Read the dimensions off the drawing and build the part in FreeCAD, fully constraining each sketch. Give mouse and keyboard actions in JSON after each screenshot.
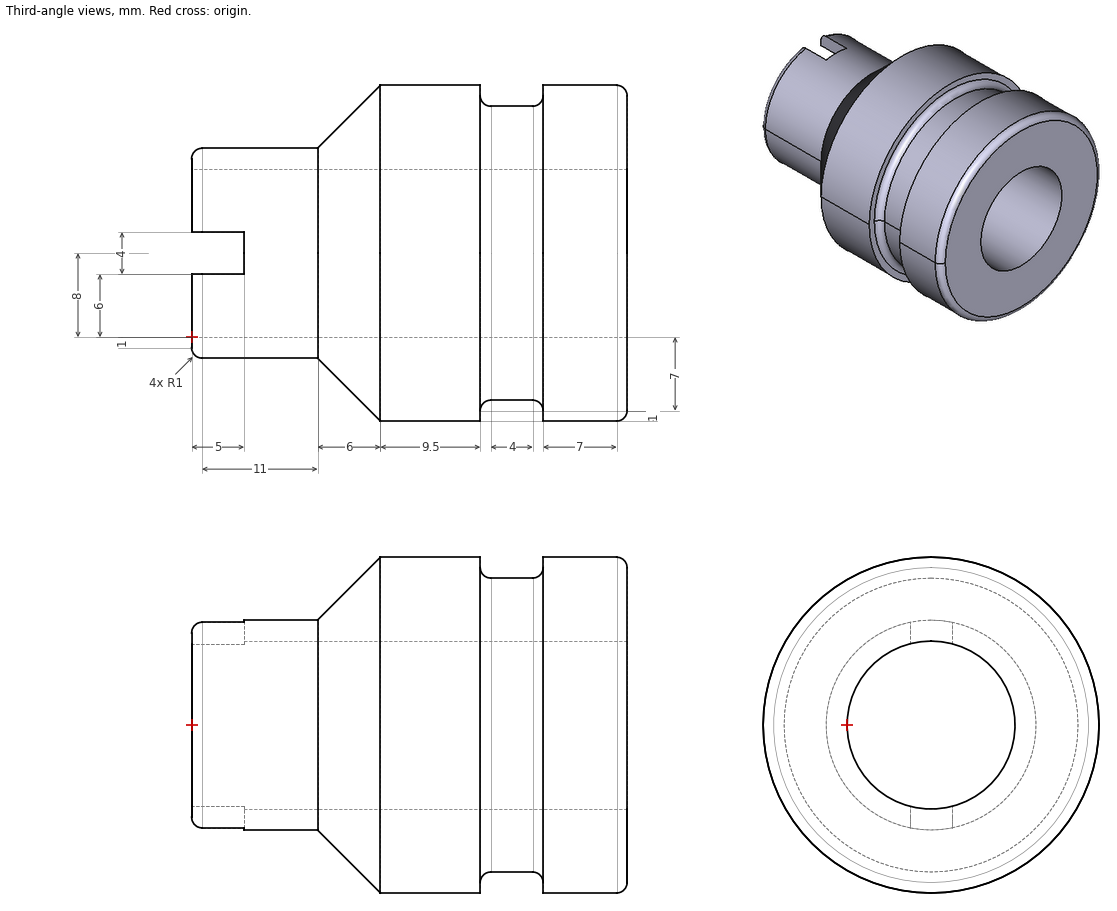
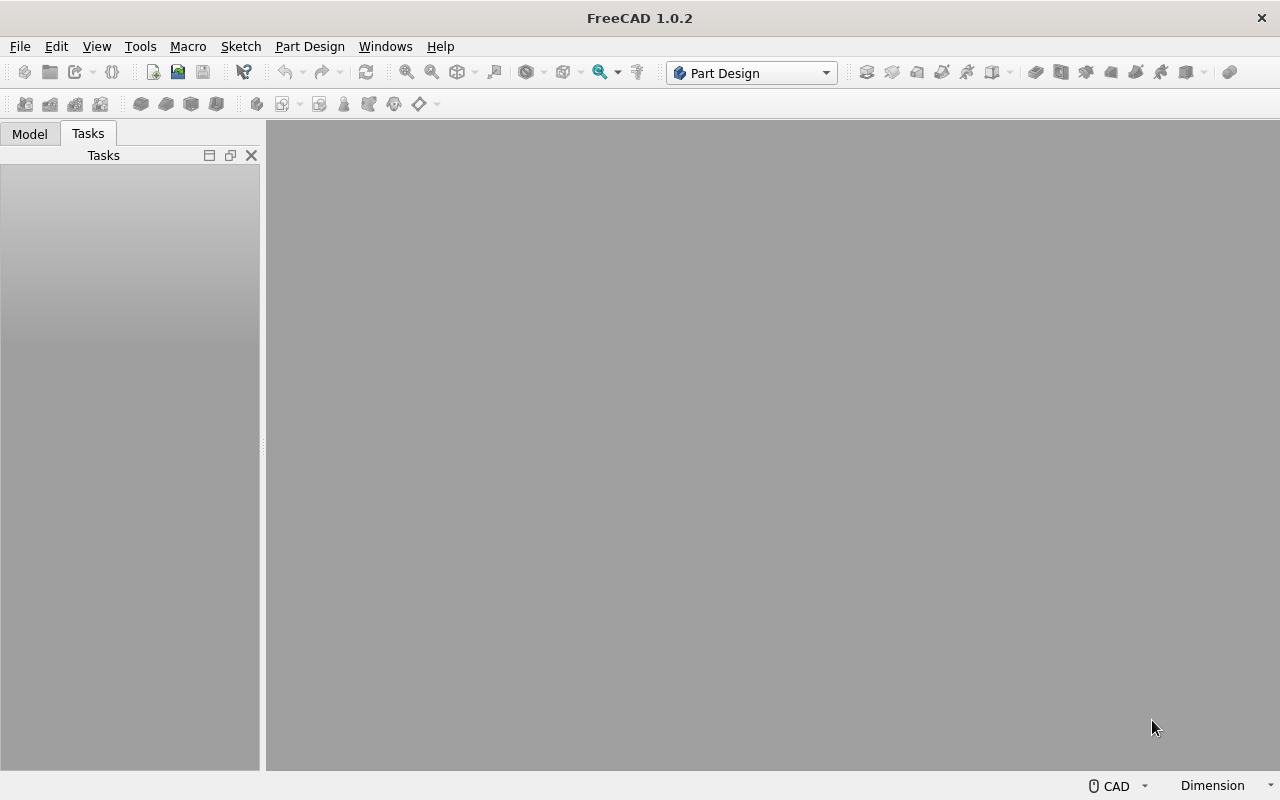
{"action": "key", "text": "ctrl+n"}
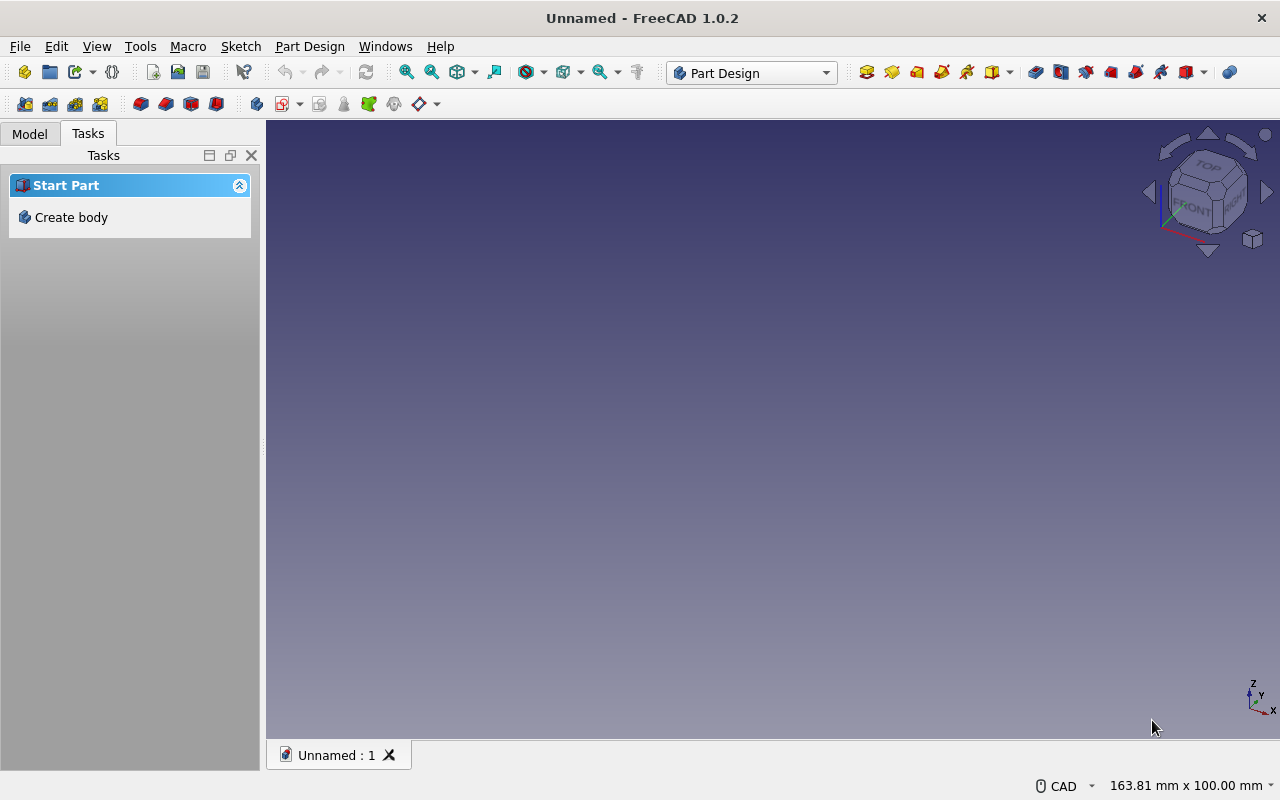
{"action": "left_click", "coordinate": [282, 104]}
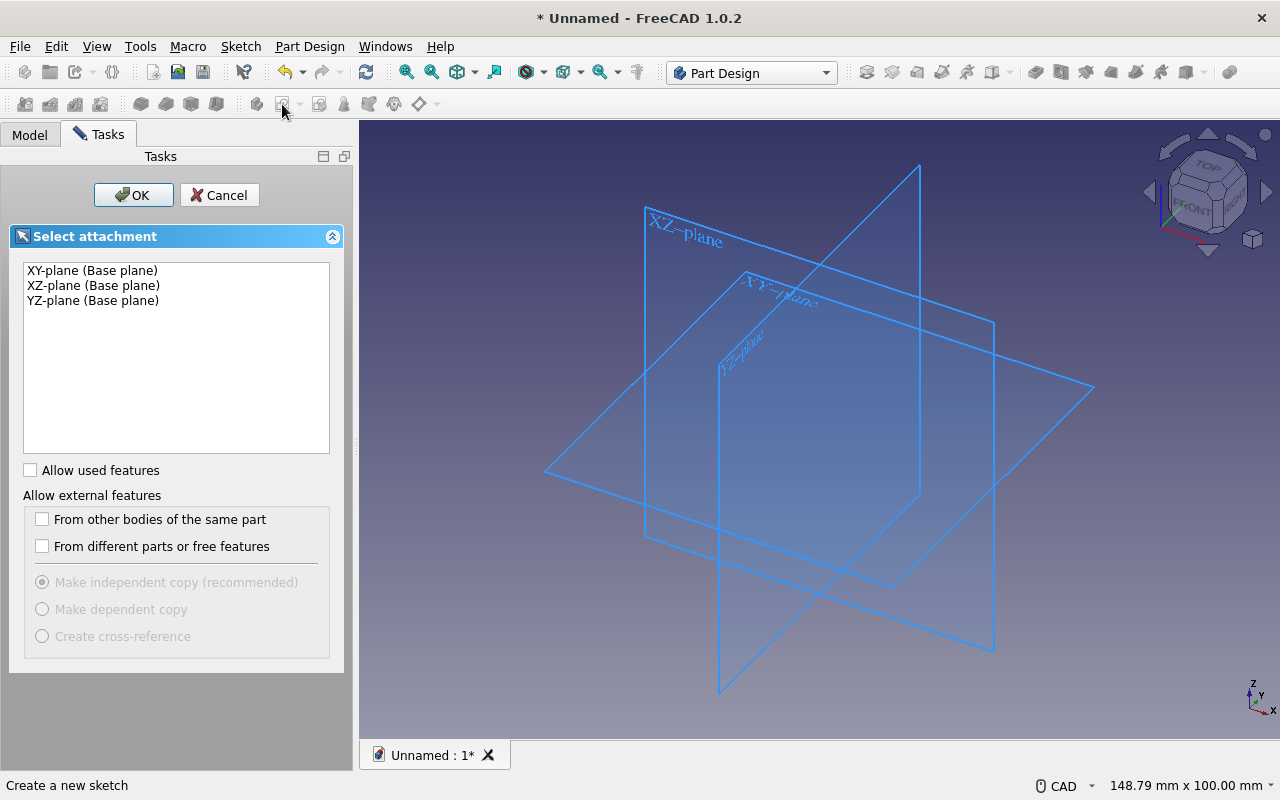
{"action": "left_click", "coordinate": [84, 270]}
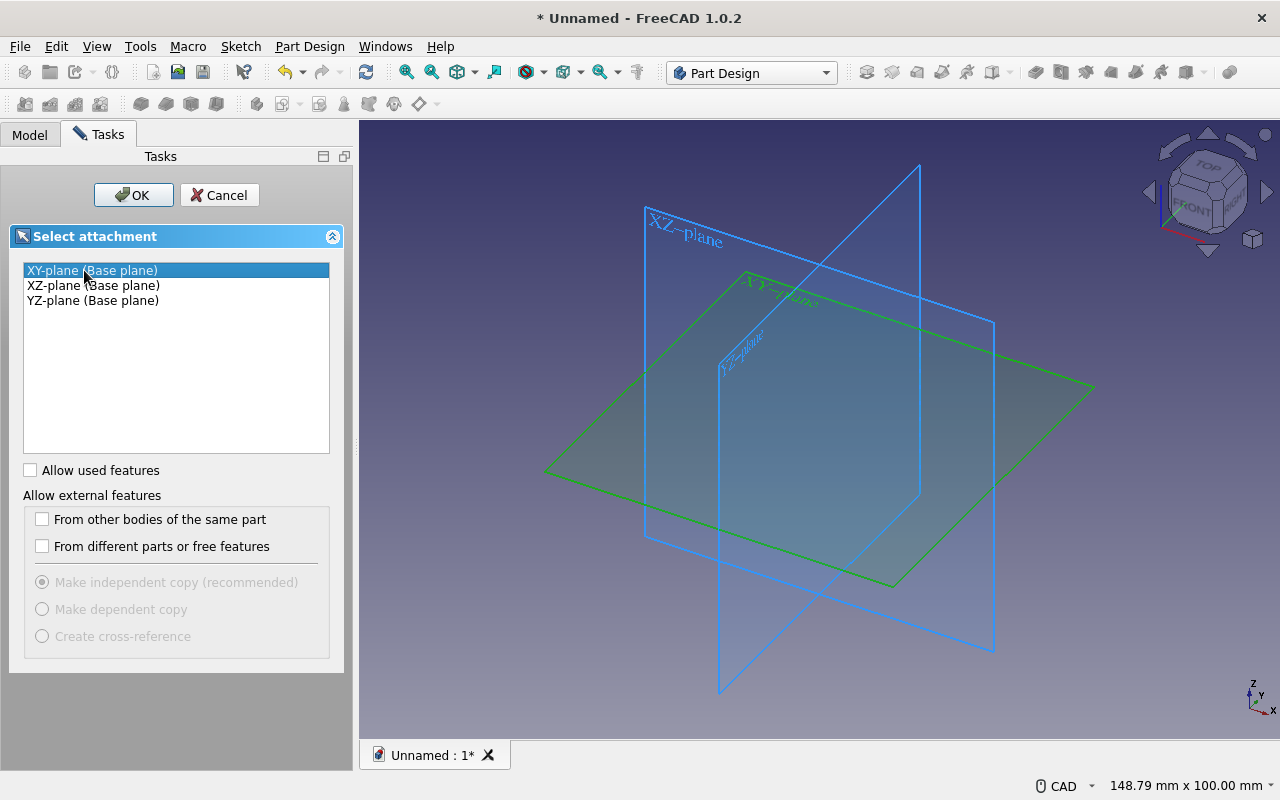
{"action": "left_click", "coordinate": [134, 195]}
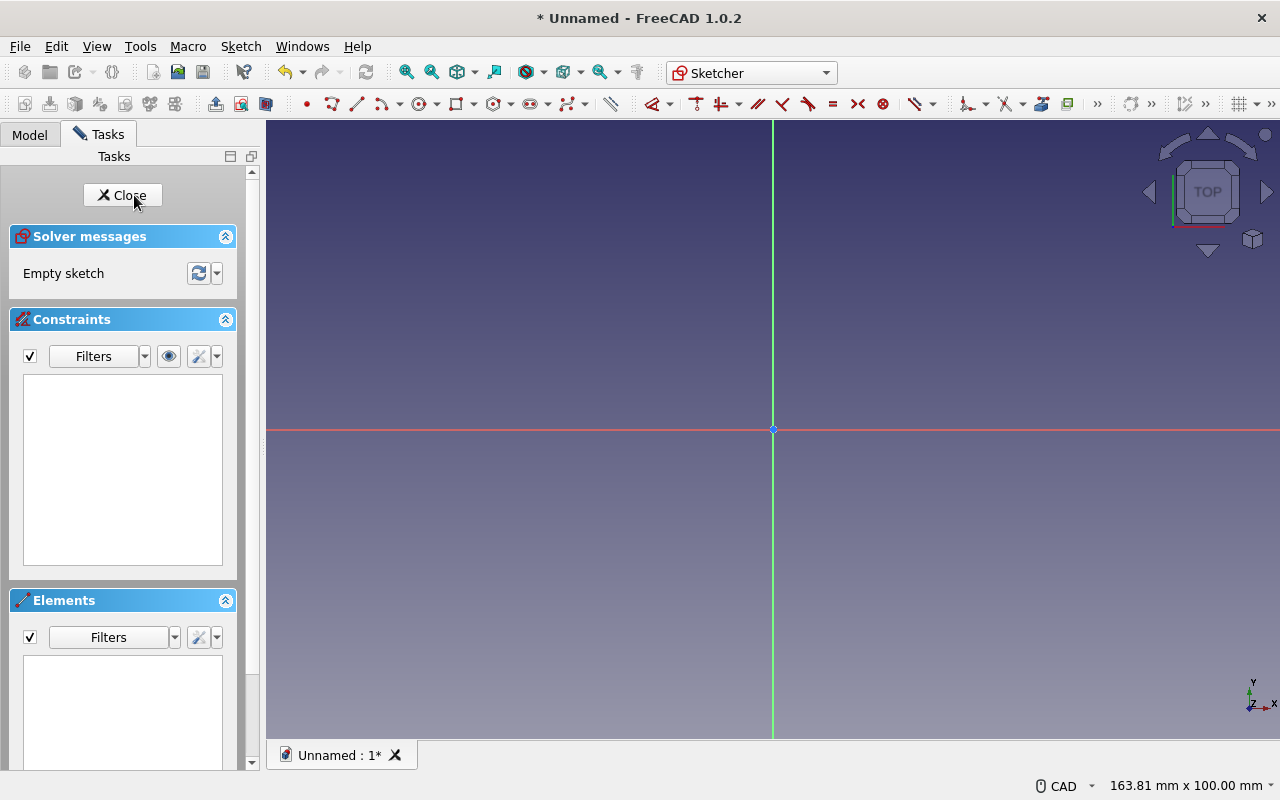
{"action": "scroll", "coordinate": [1115, 430], "scroll_direction": "up", "scroll_amount": 3}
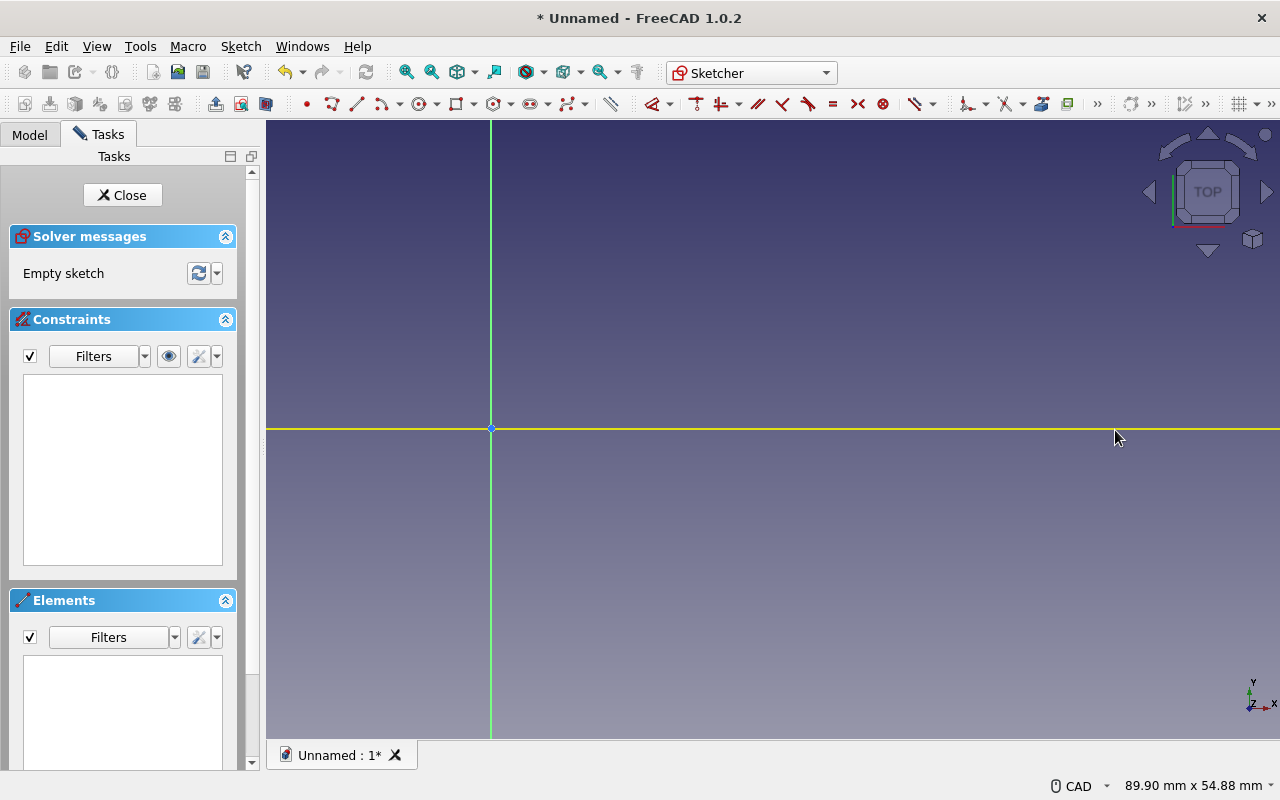
{"action": "left_click", "coordinate": [332, 104]}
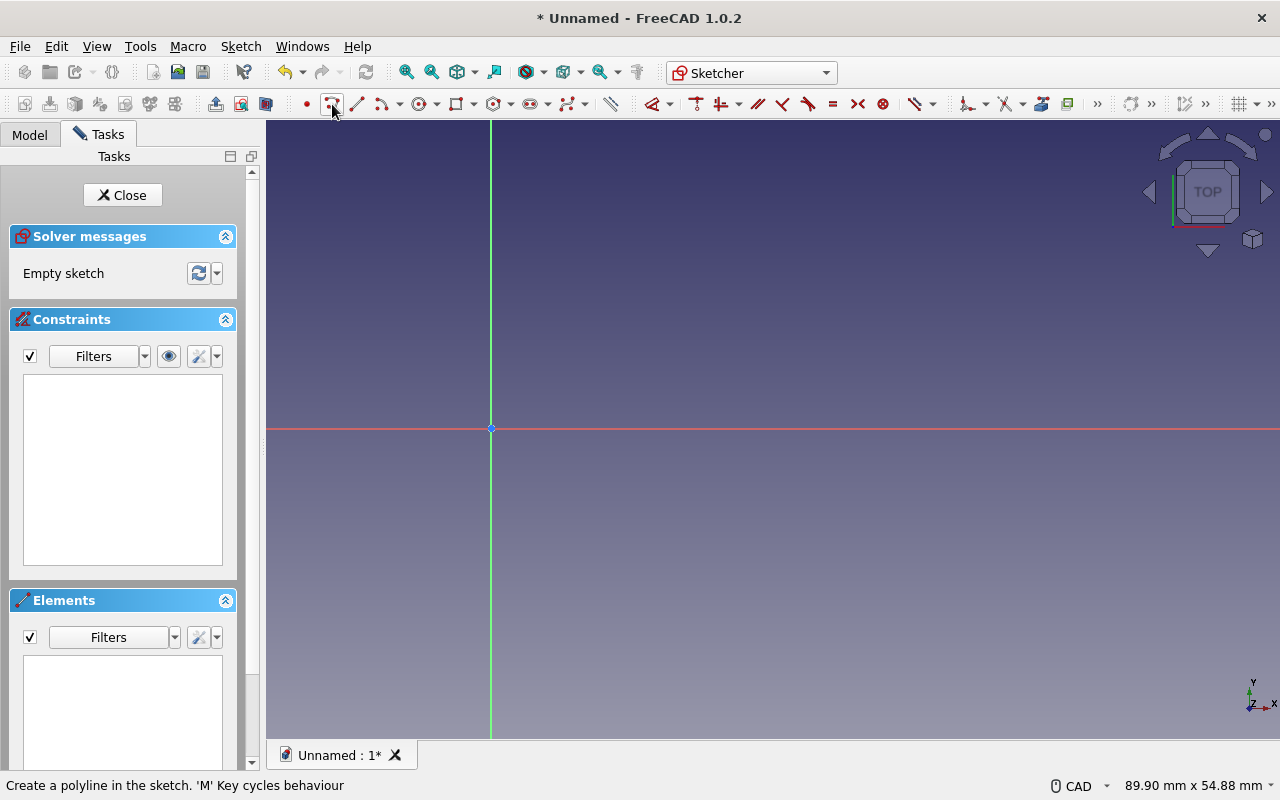
{"action": "scroll", "coordinate": [502, 451], "scroll_direction": "up", "scroll_amount": 2}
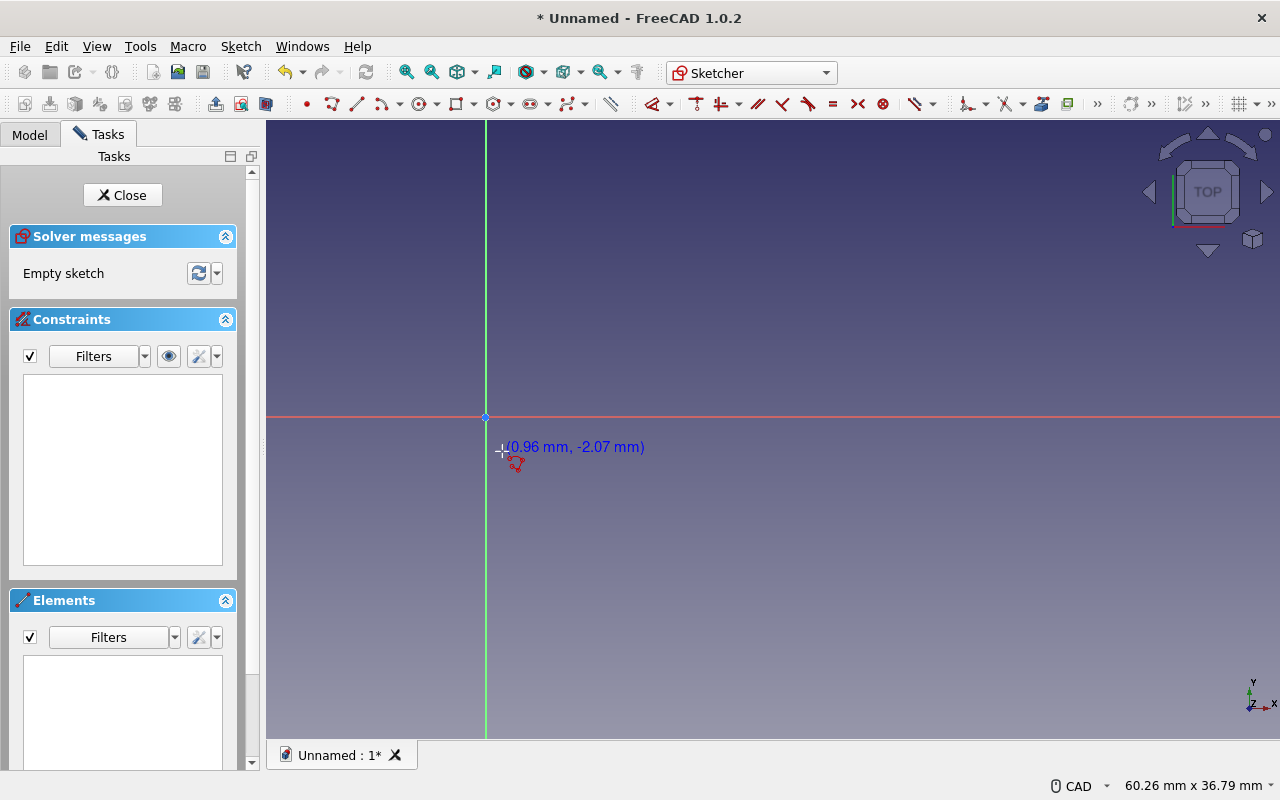
{"action": "left_click", "coordinate": [503, 451]}
{"action": "left_click", "coordinate": [688, 451]}
{"action": "left_click", "coordinate": [789, 552]}
{"action": "left_click", "coordinate": [948, 552]}
{"action": "left_click", "coordinate": [948, 535]}
{"action": "right_click", "coordinate": [948, 535]}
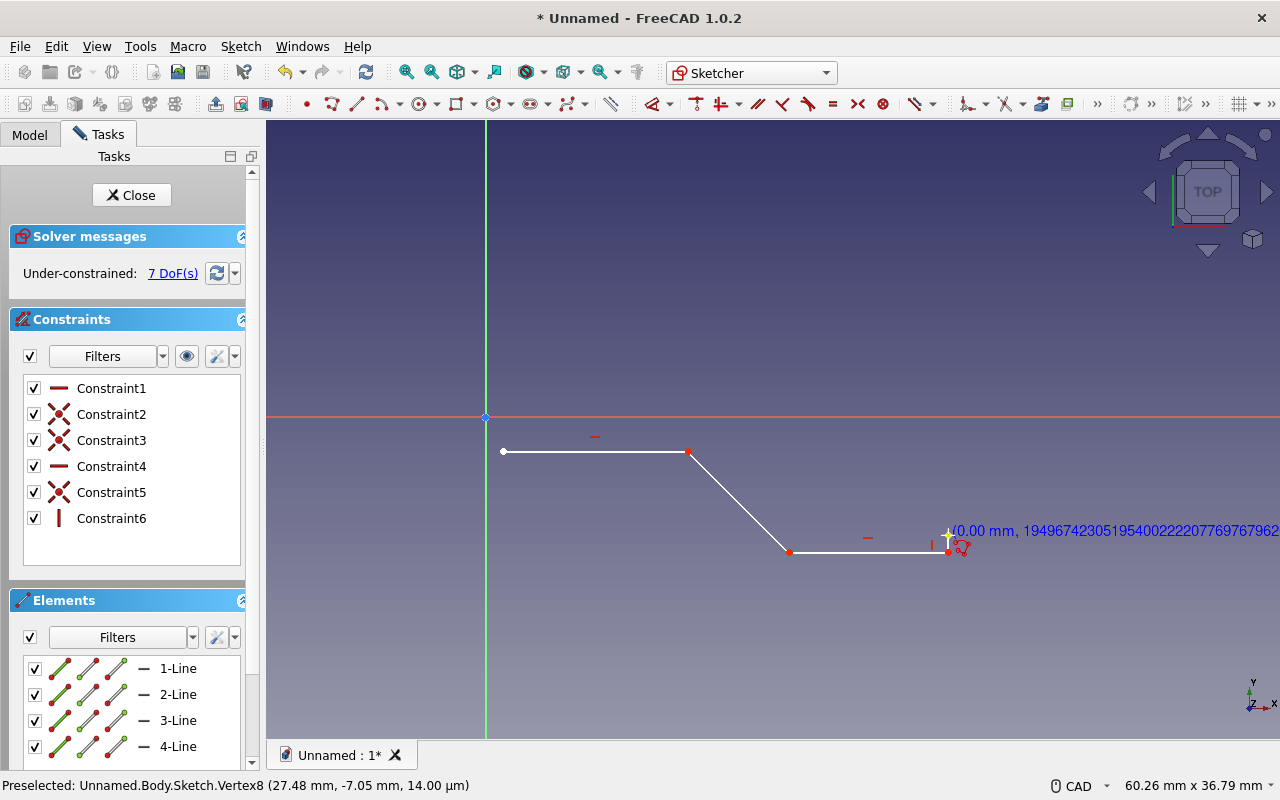
{"action": "key", "text": "g l"}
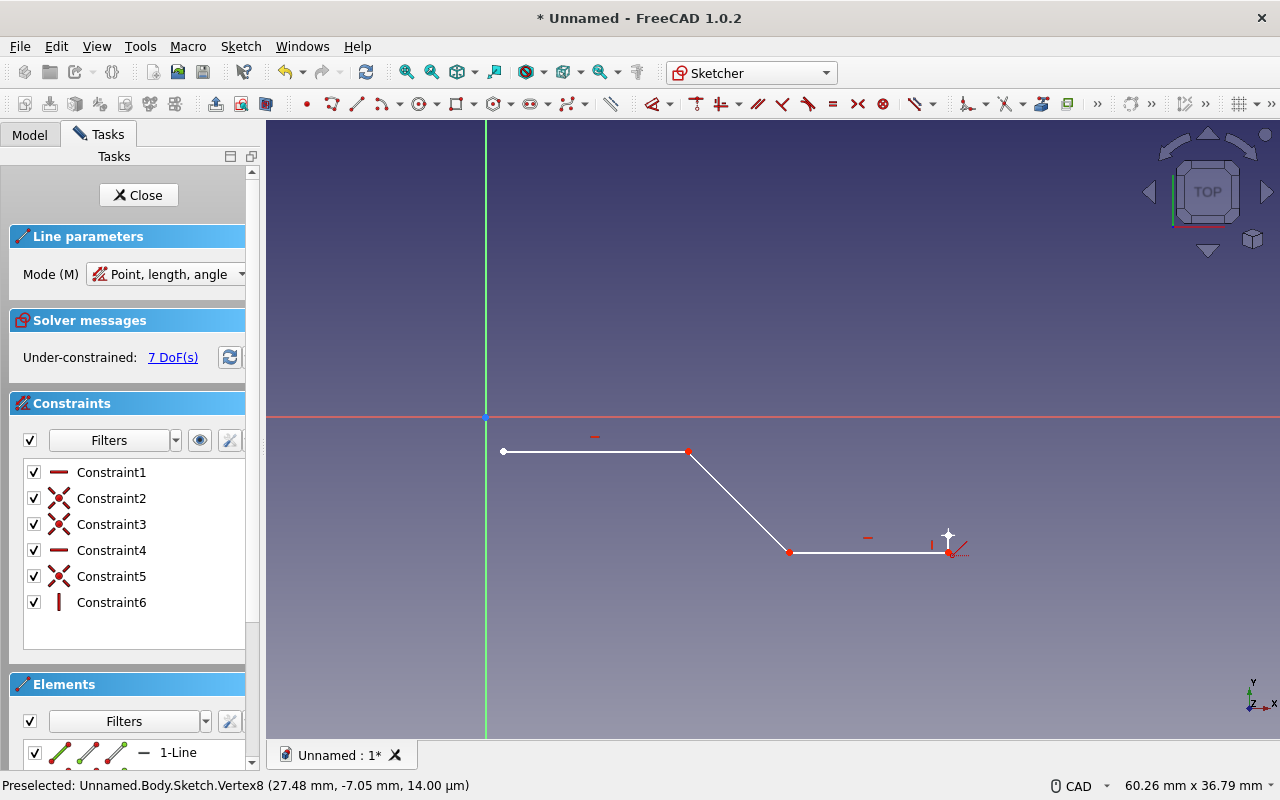
{"action": "left_click", "coordinate": [965, 518]}
{"action": "left_click", "coordinate": [1033, 518]}